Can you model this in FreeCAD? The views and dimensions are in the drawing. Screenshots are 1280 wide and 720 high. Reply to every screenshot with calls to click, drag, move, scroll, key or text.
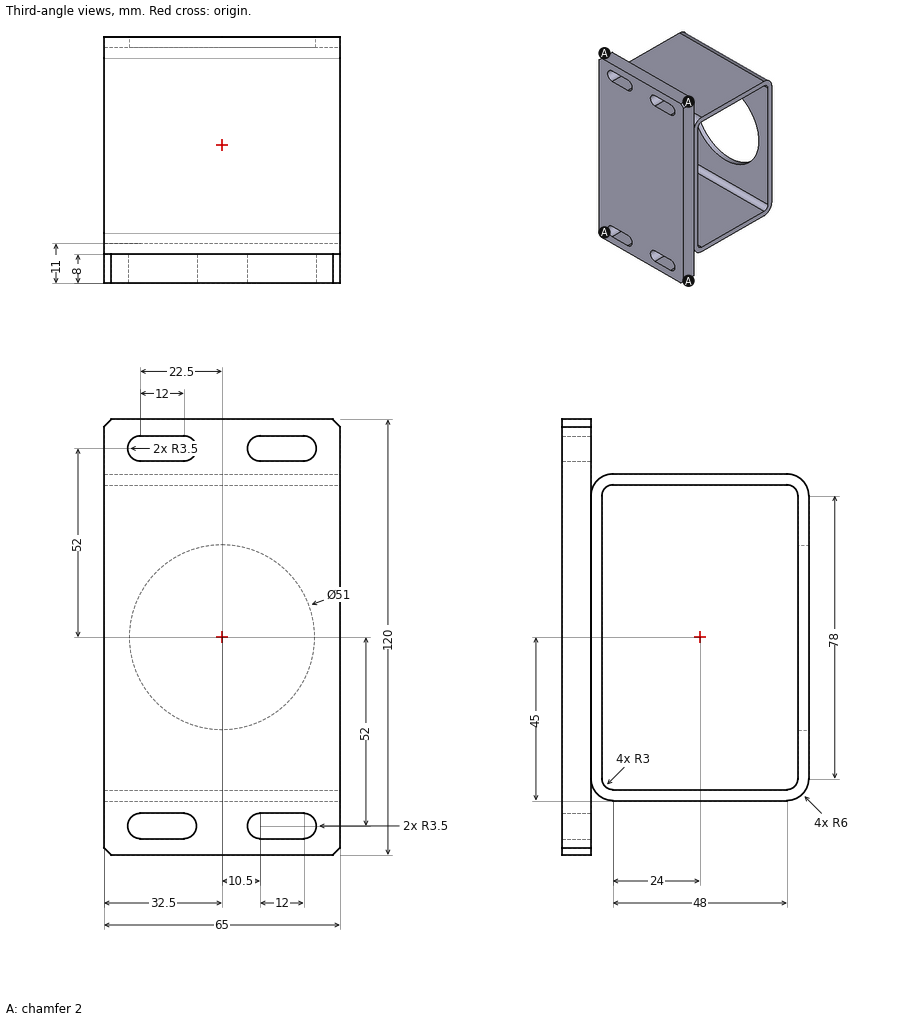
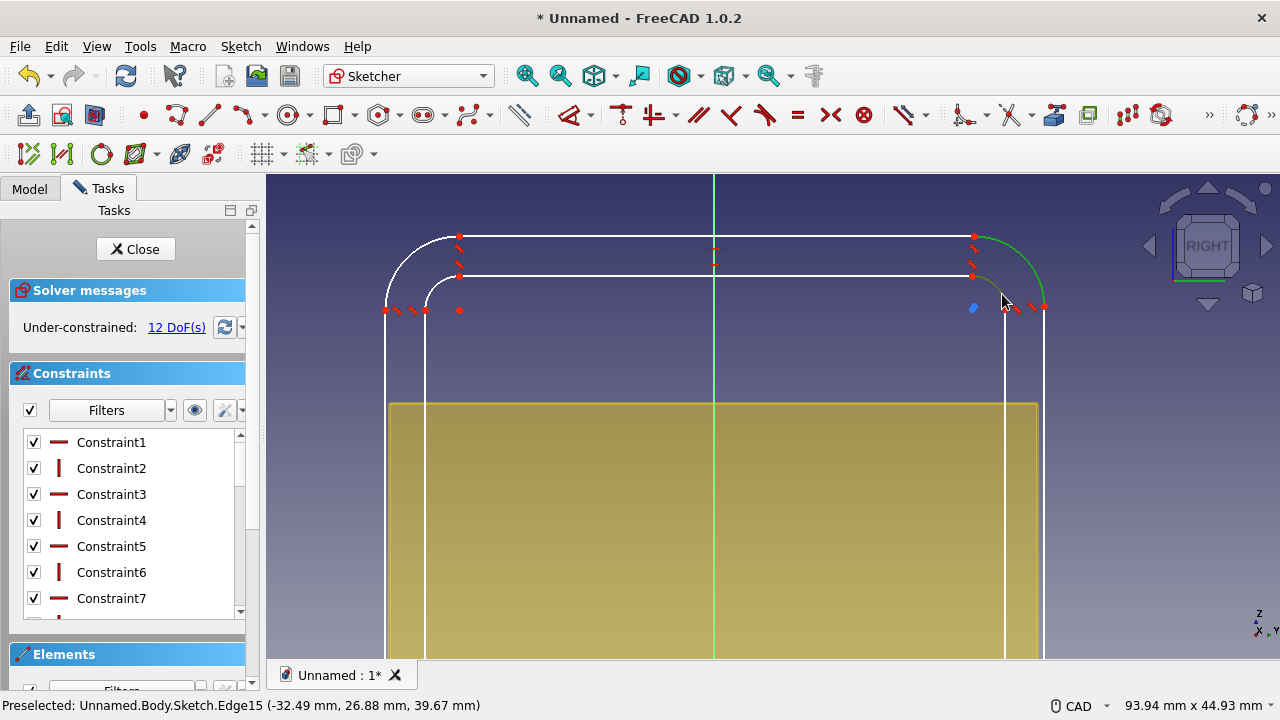
click(621, 116)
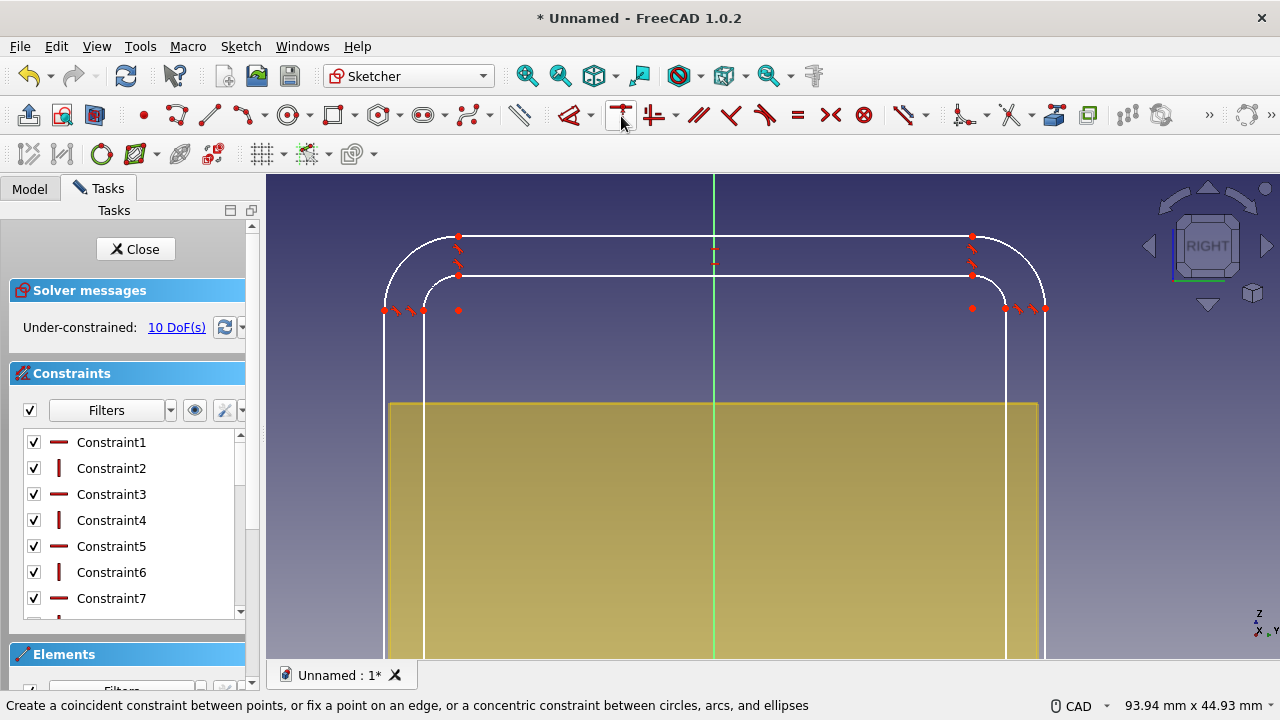
scroll(701, 283, down, 6)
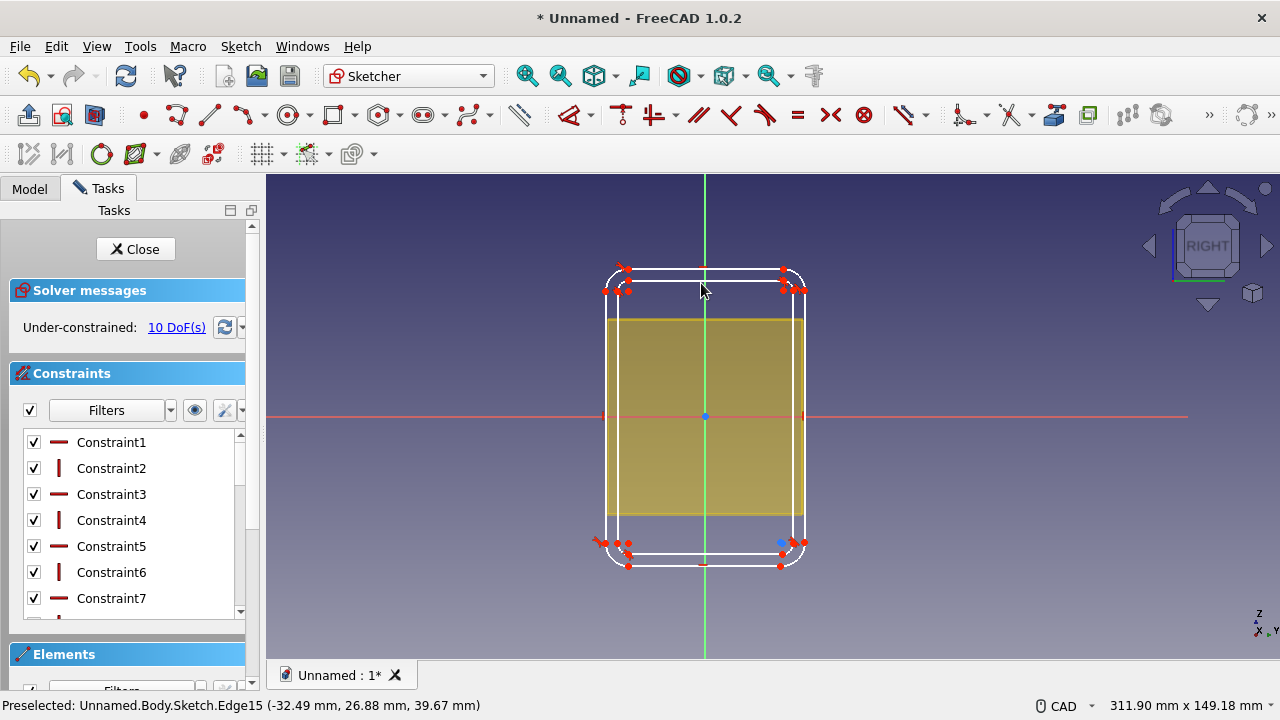
scroll(792, 564, up, 2)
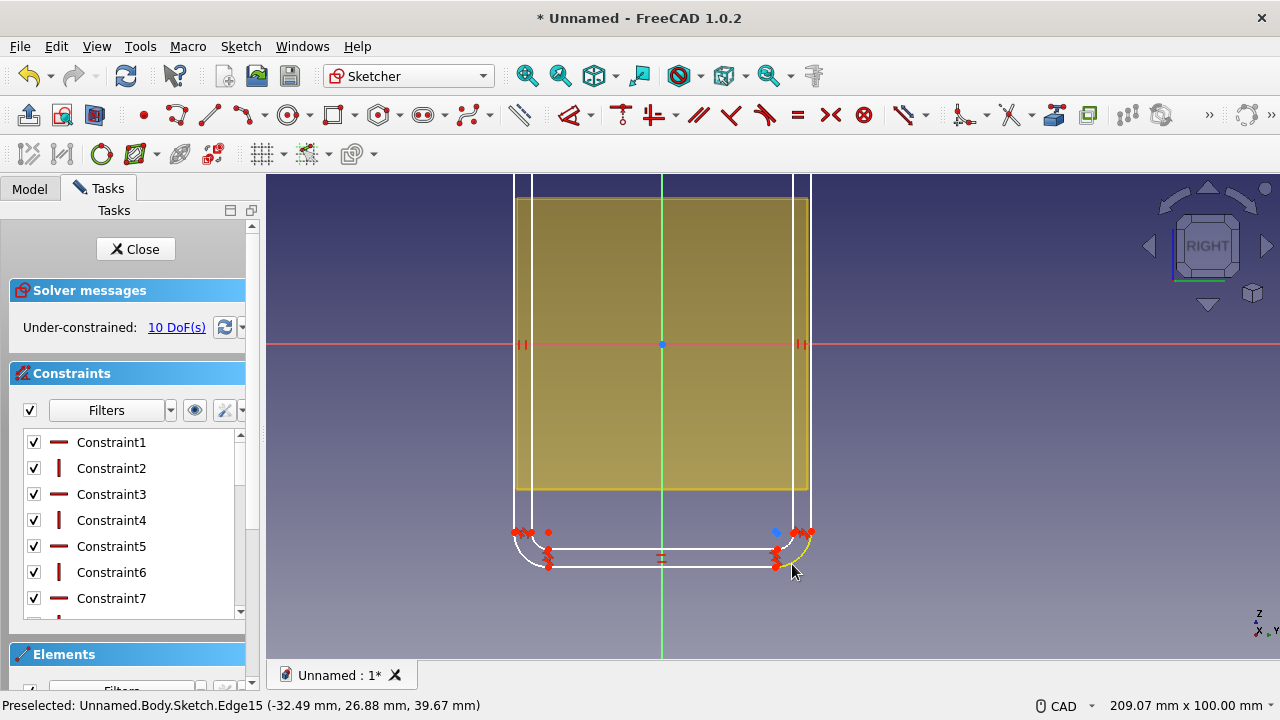
click(792, 563)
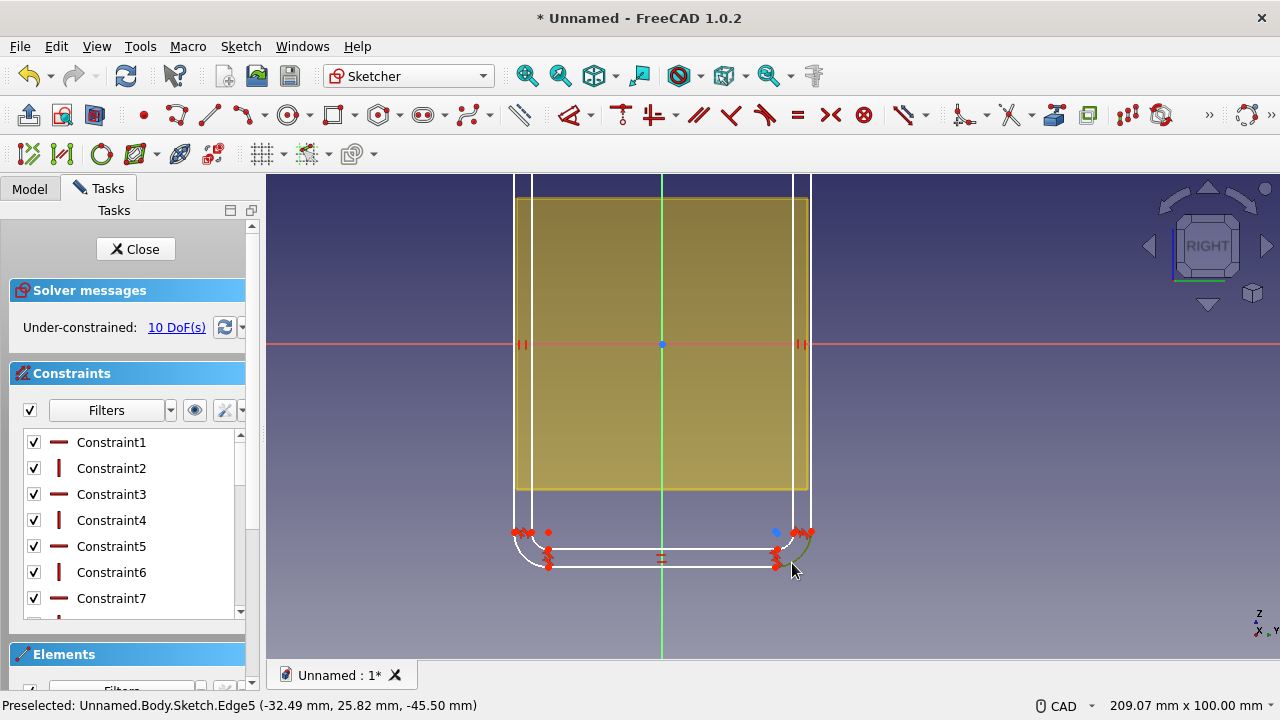
scroll(791, 564, down, 2)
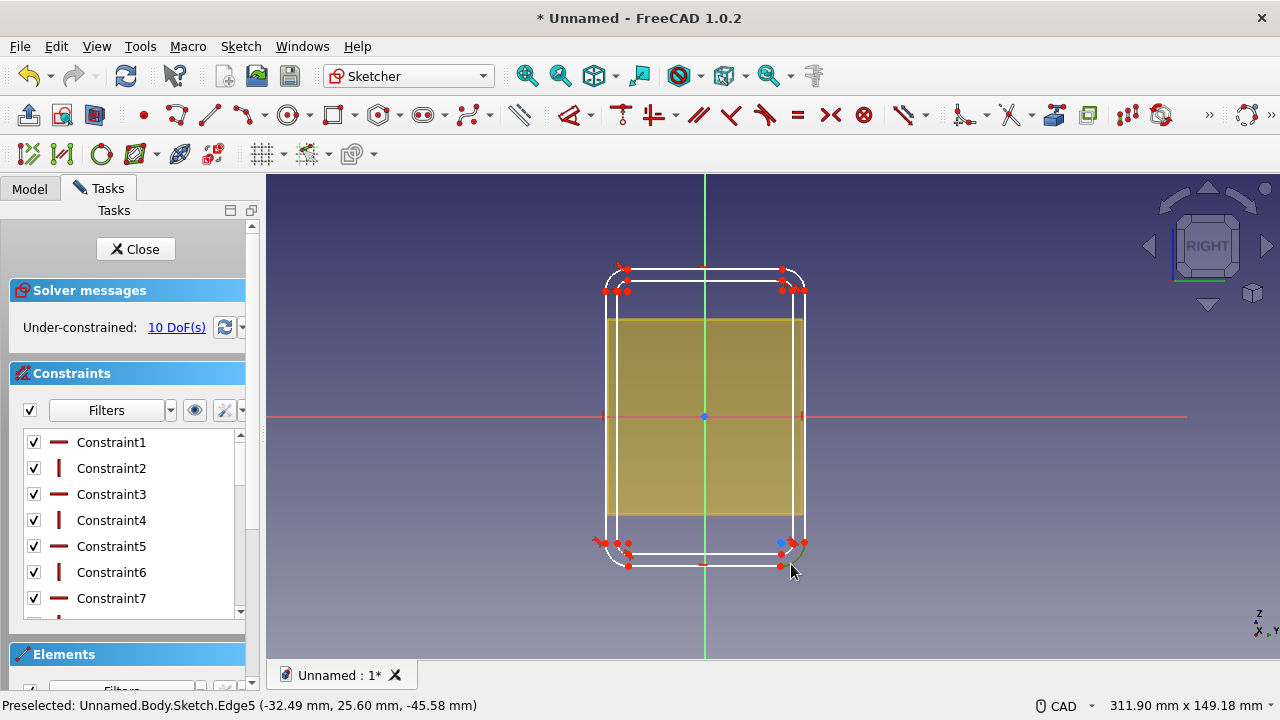
scroll(802, 281, up, 2)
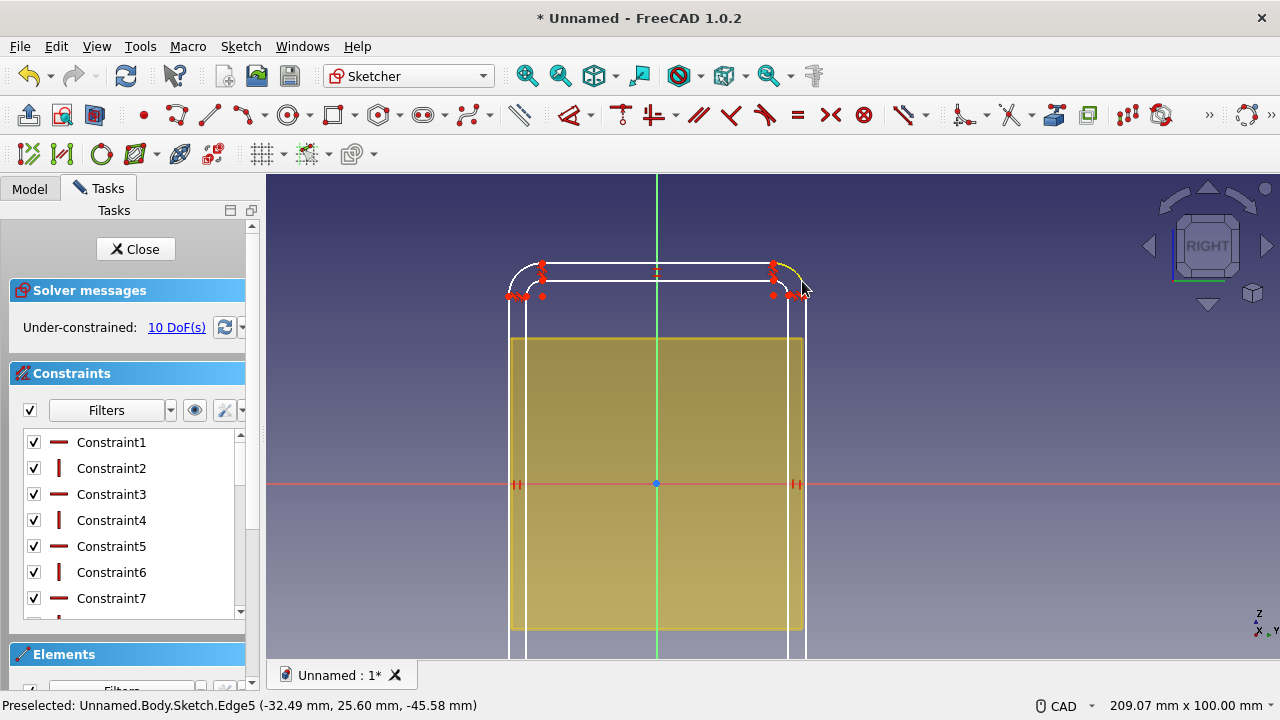
click(802, 281)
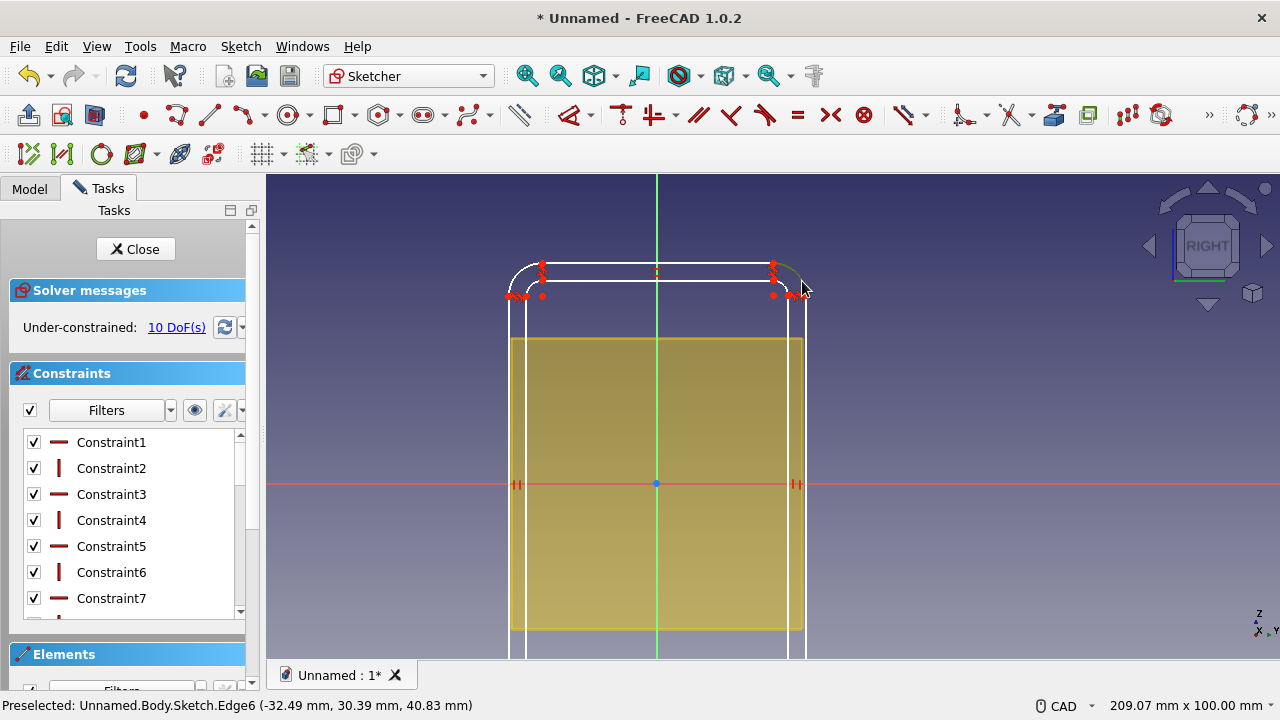
click(527, 267)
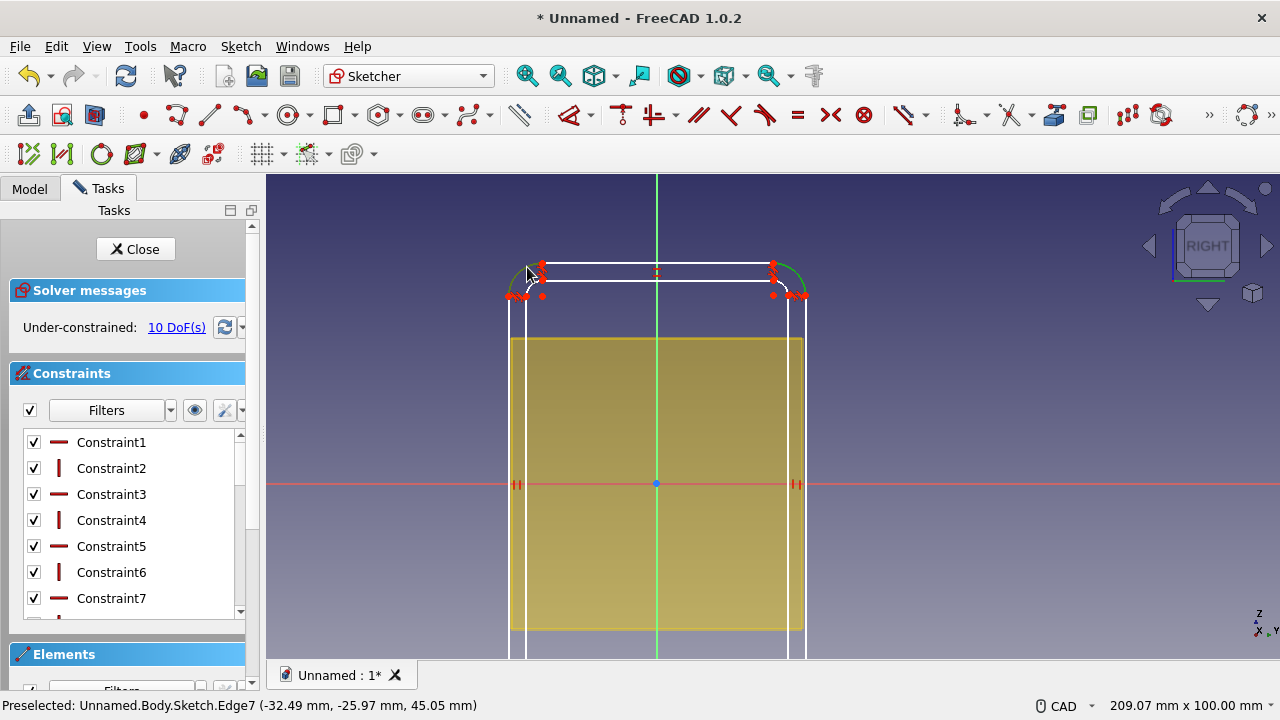
scroll(802, 280, down, 2)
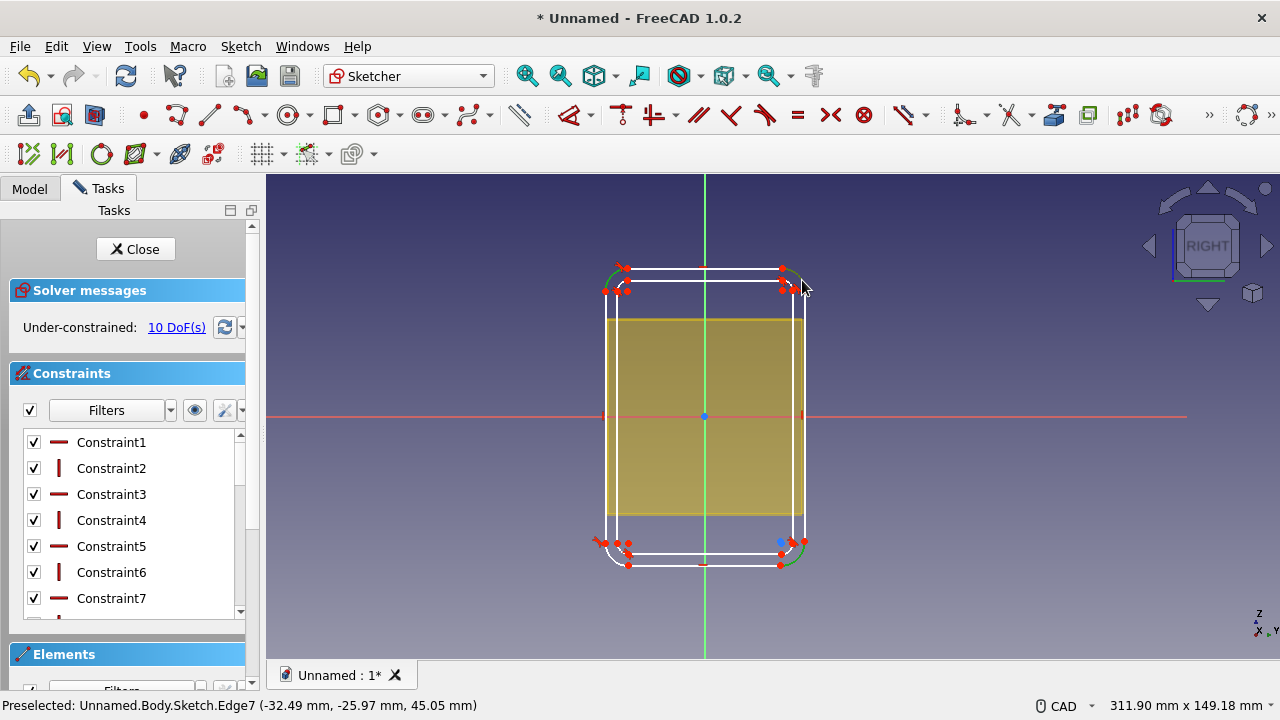
scroll(608, 553, up, 2)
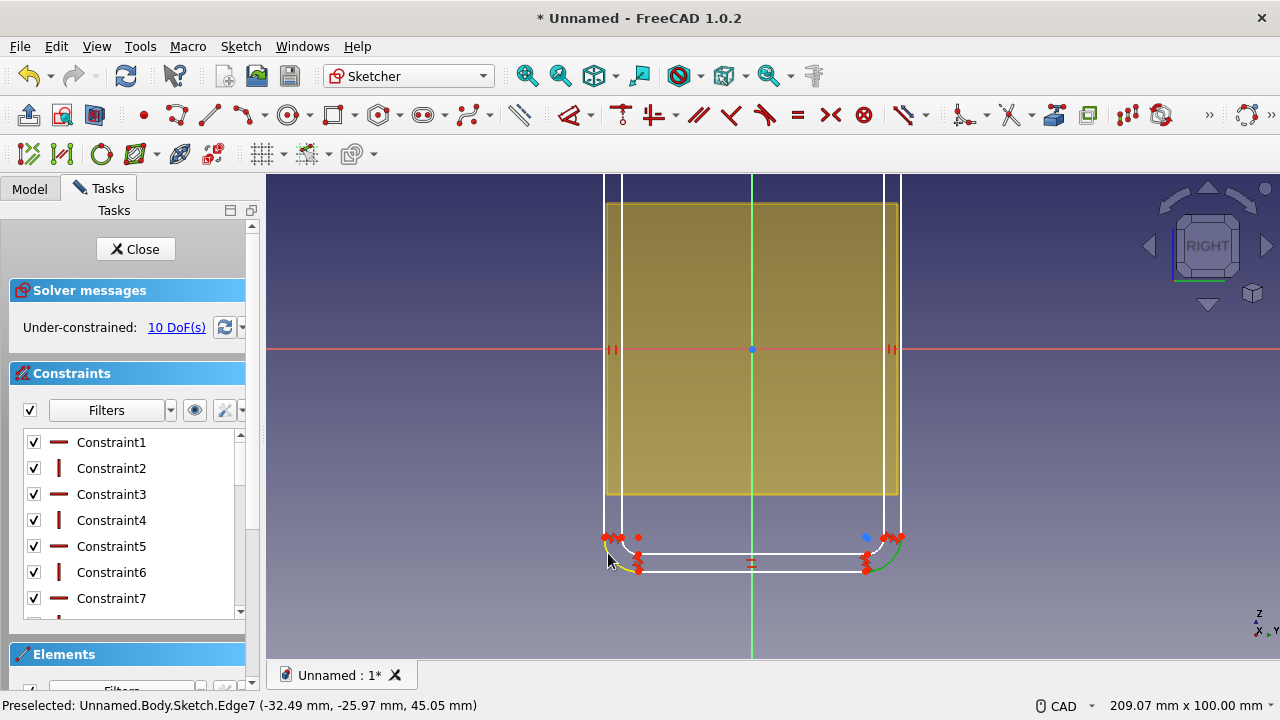
click(608, 553)